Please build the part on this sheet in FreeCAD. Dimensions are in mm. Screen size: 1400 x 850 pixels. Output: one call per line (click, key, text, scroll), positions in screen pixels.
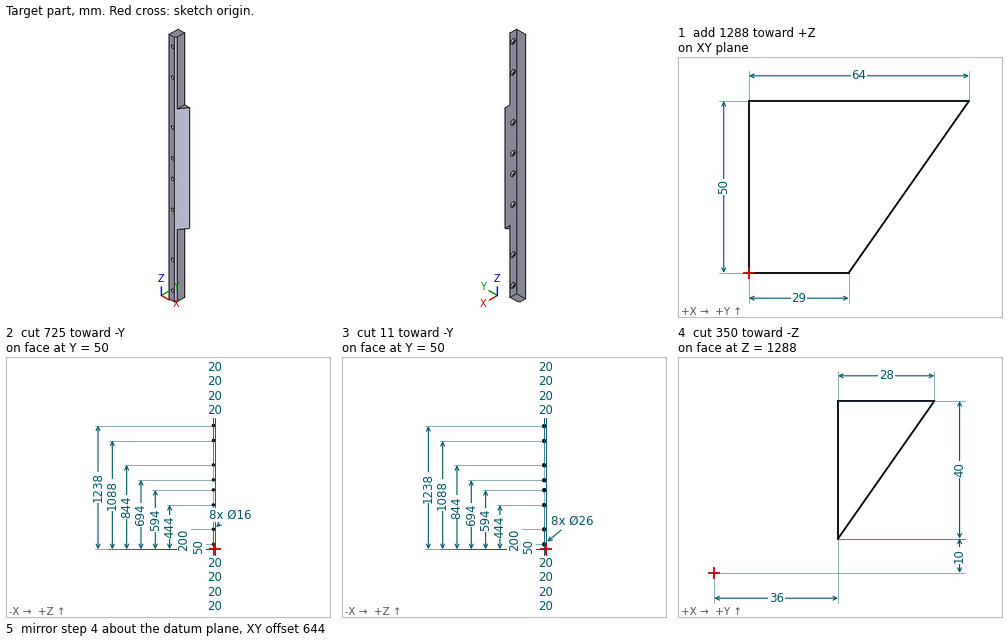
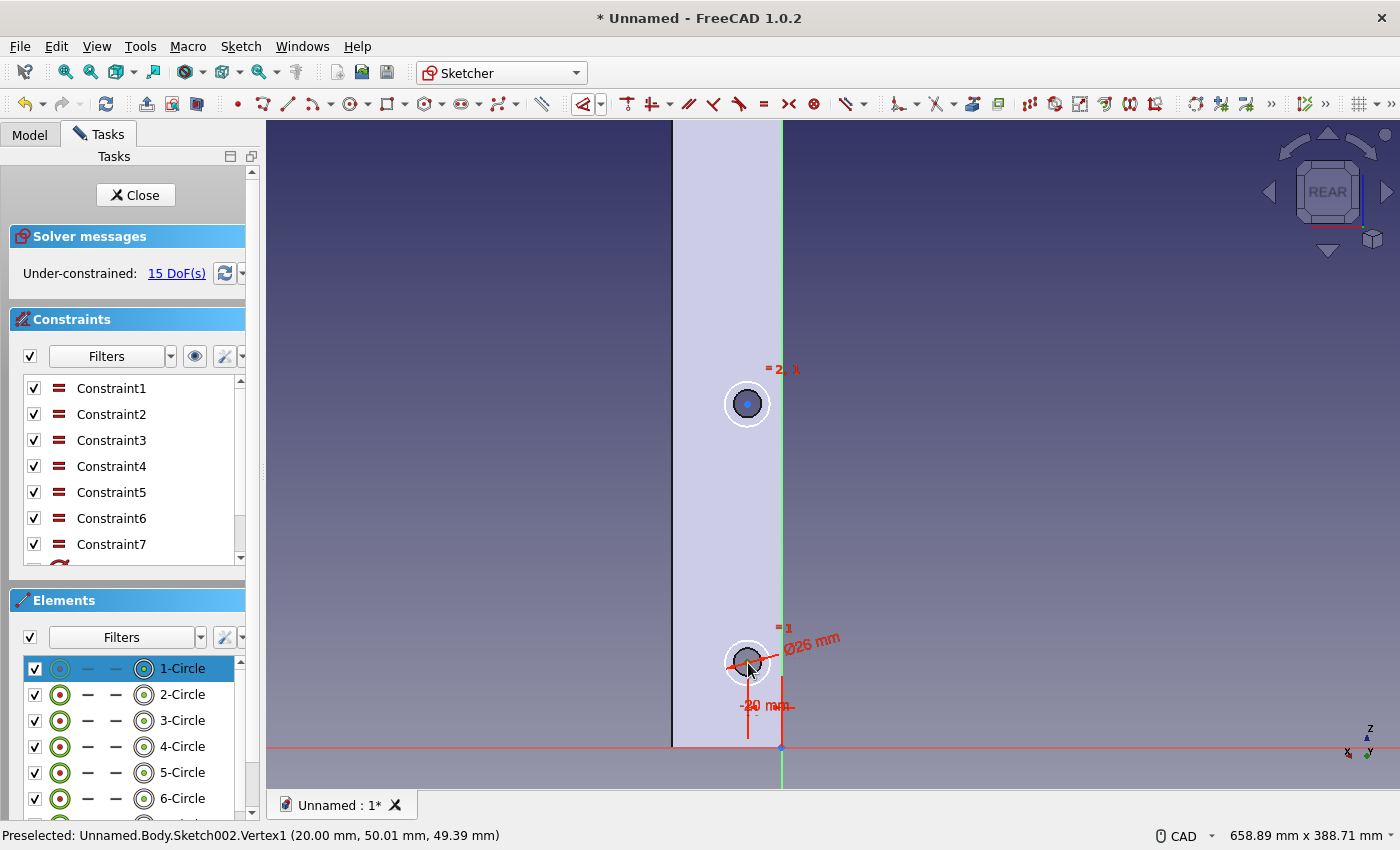
key(i)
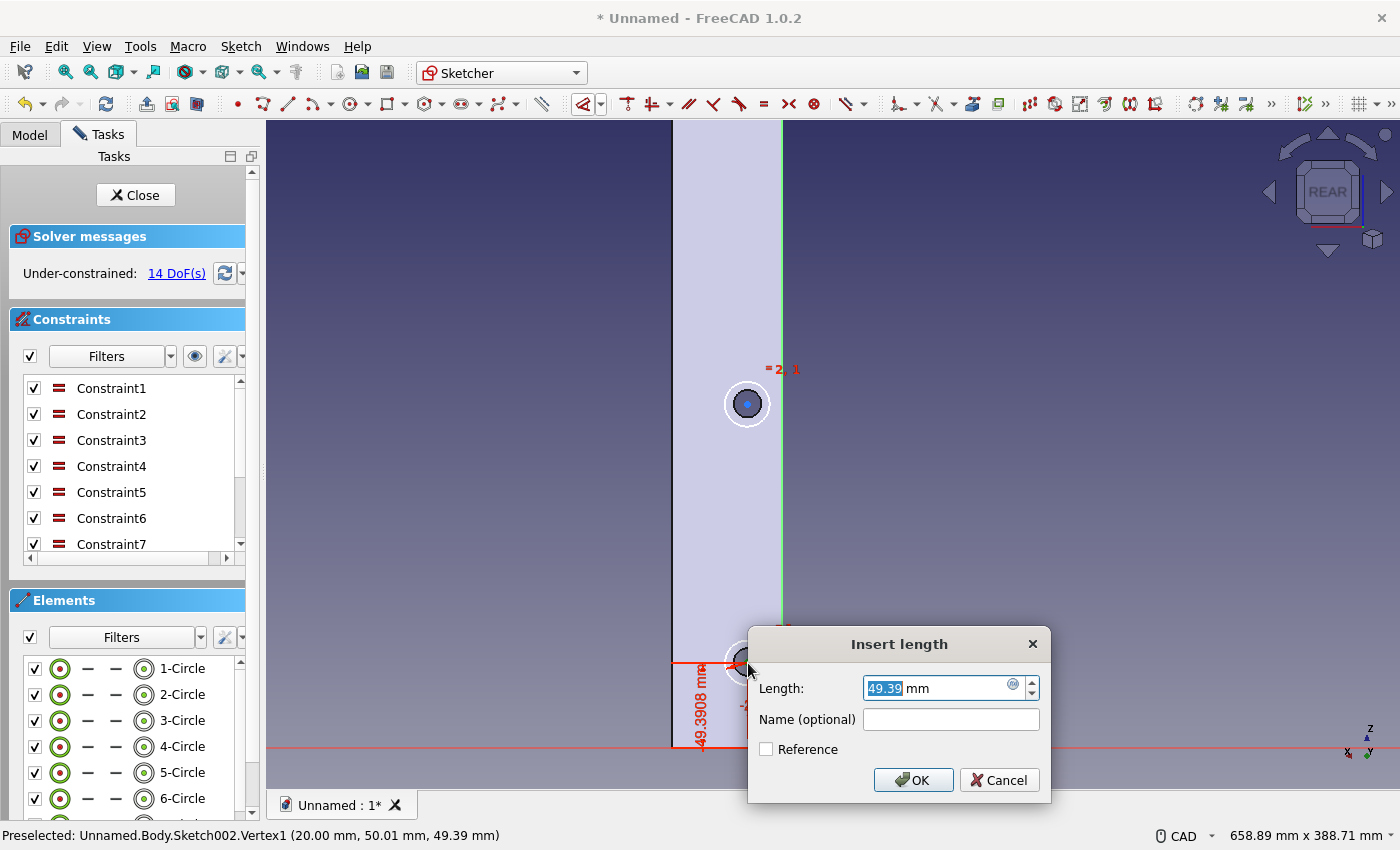
text(50)
key(Return)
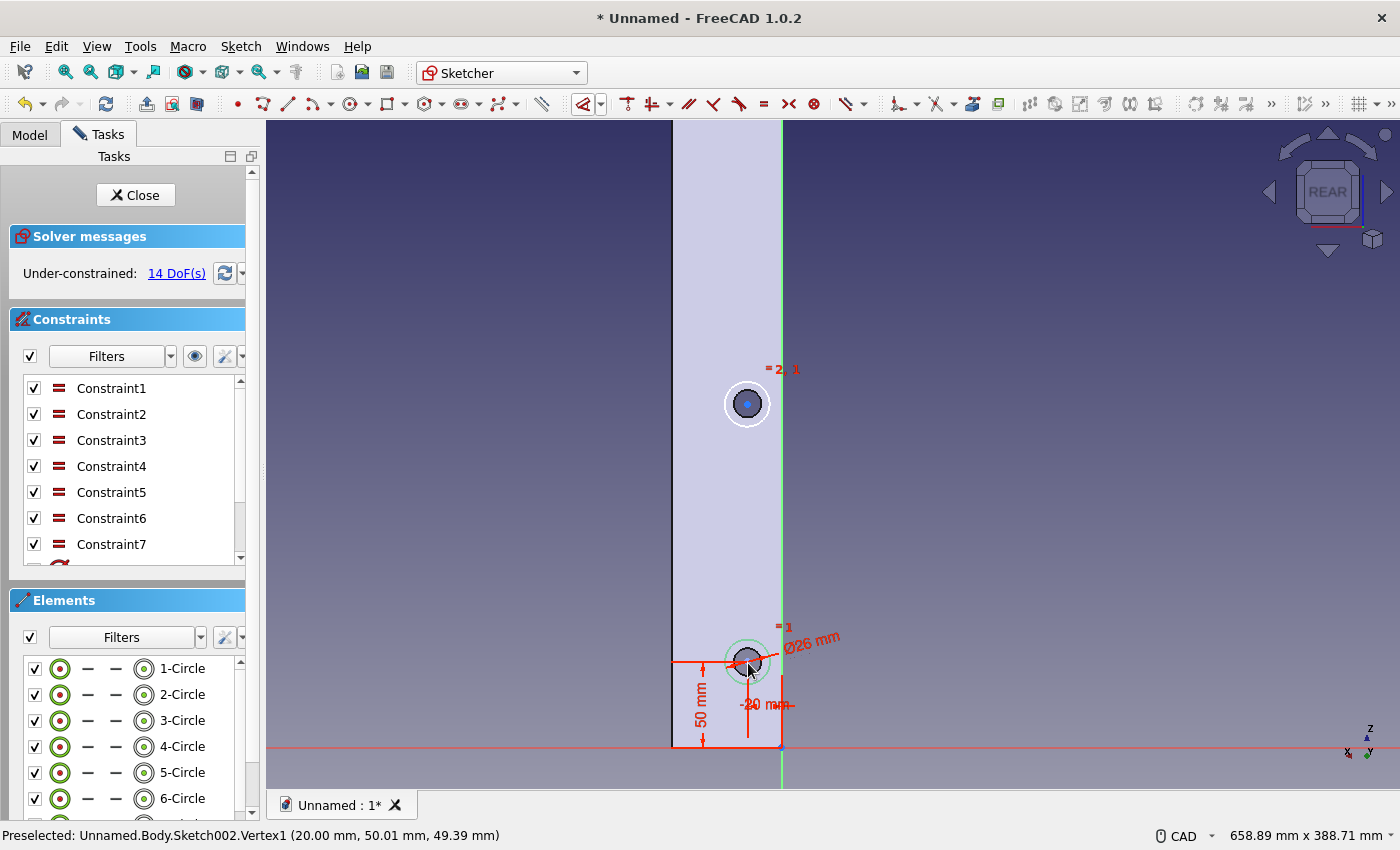
click(747, 404)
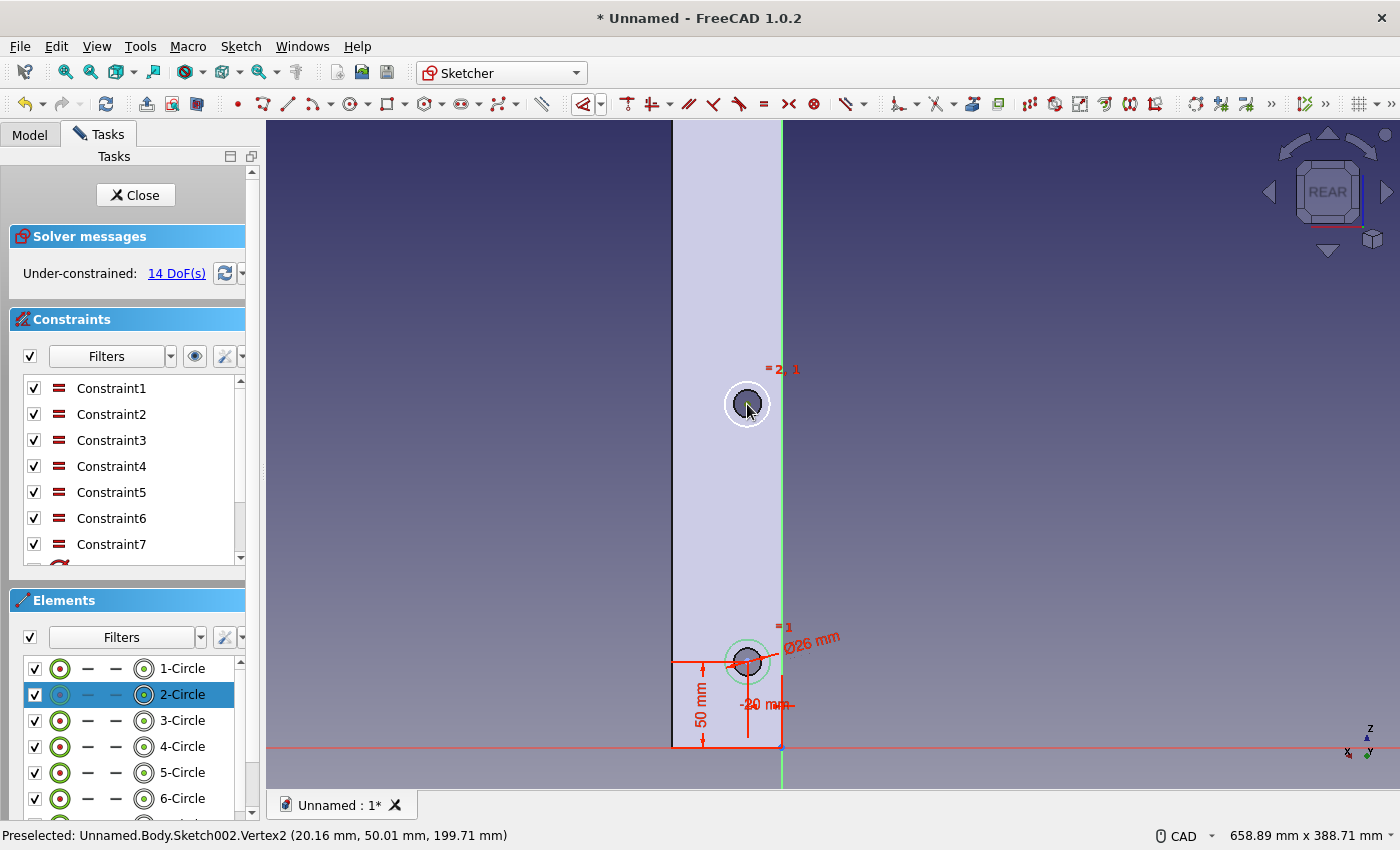
key(l)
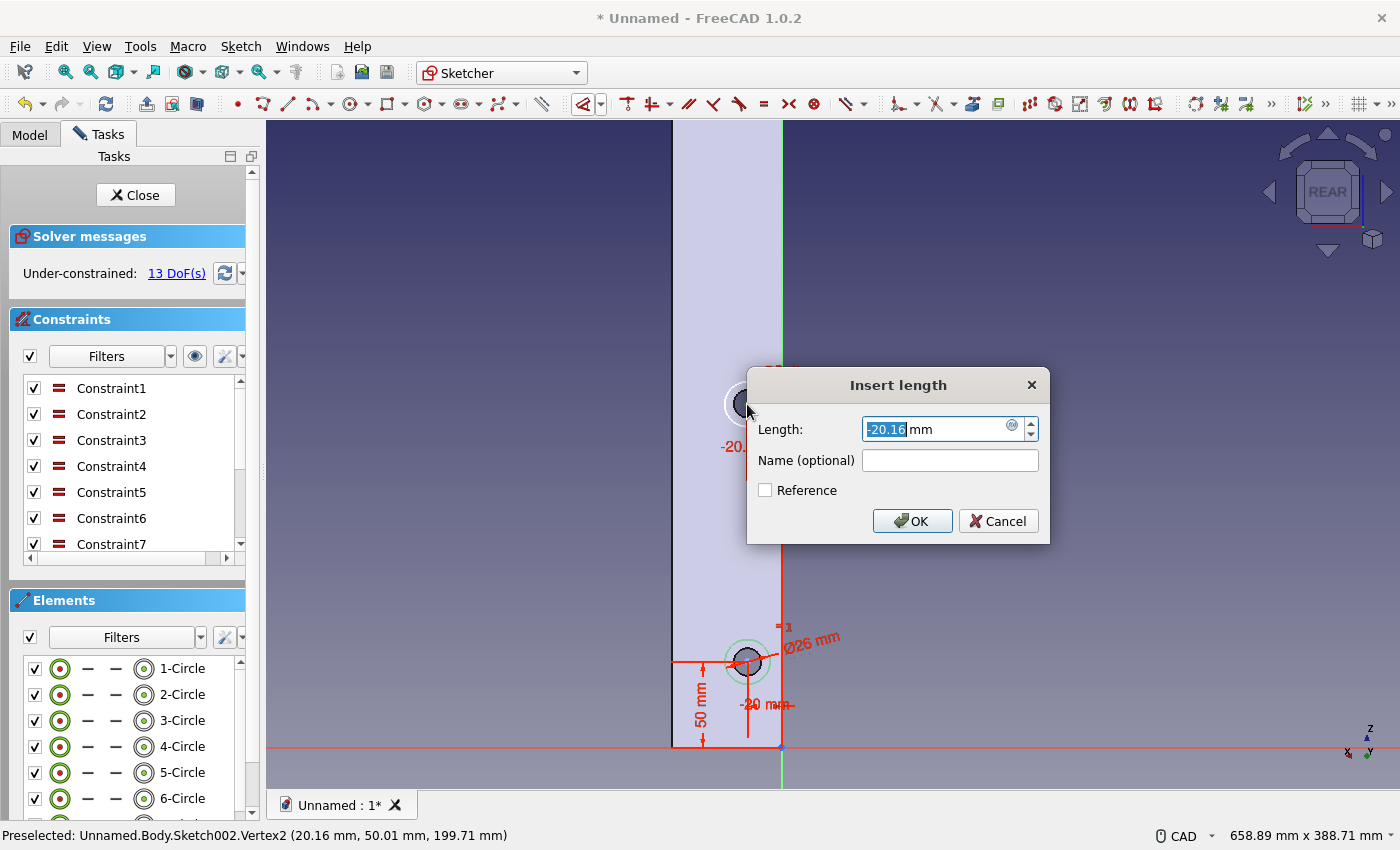
text(-20)
key(Return)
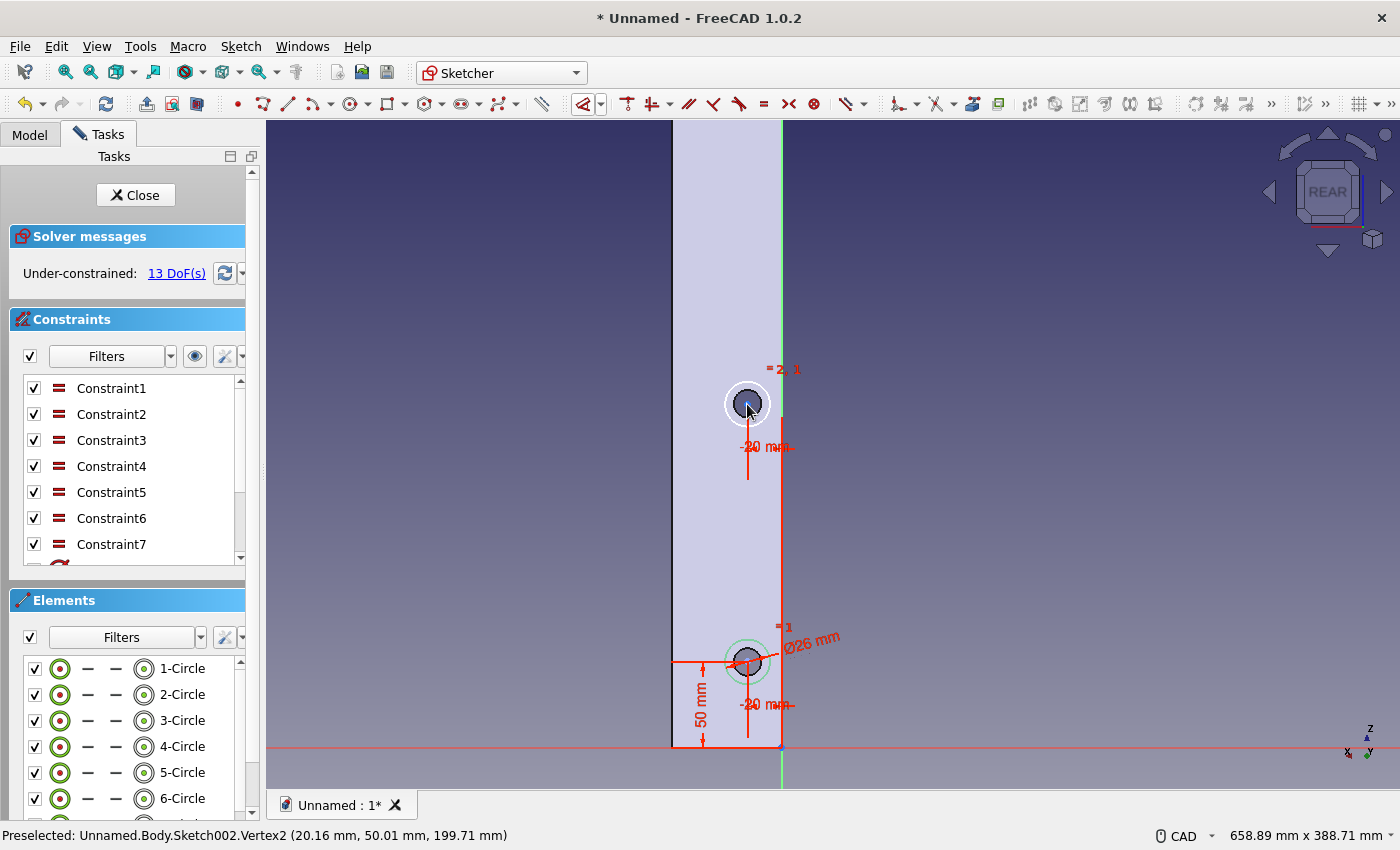
scroll(767, 653, down, 8)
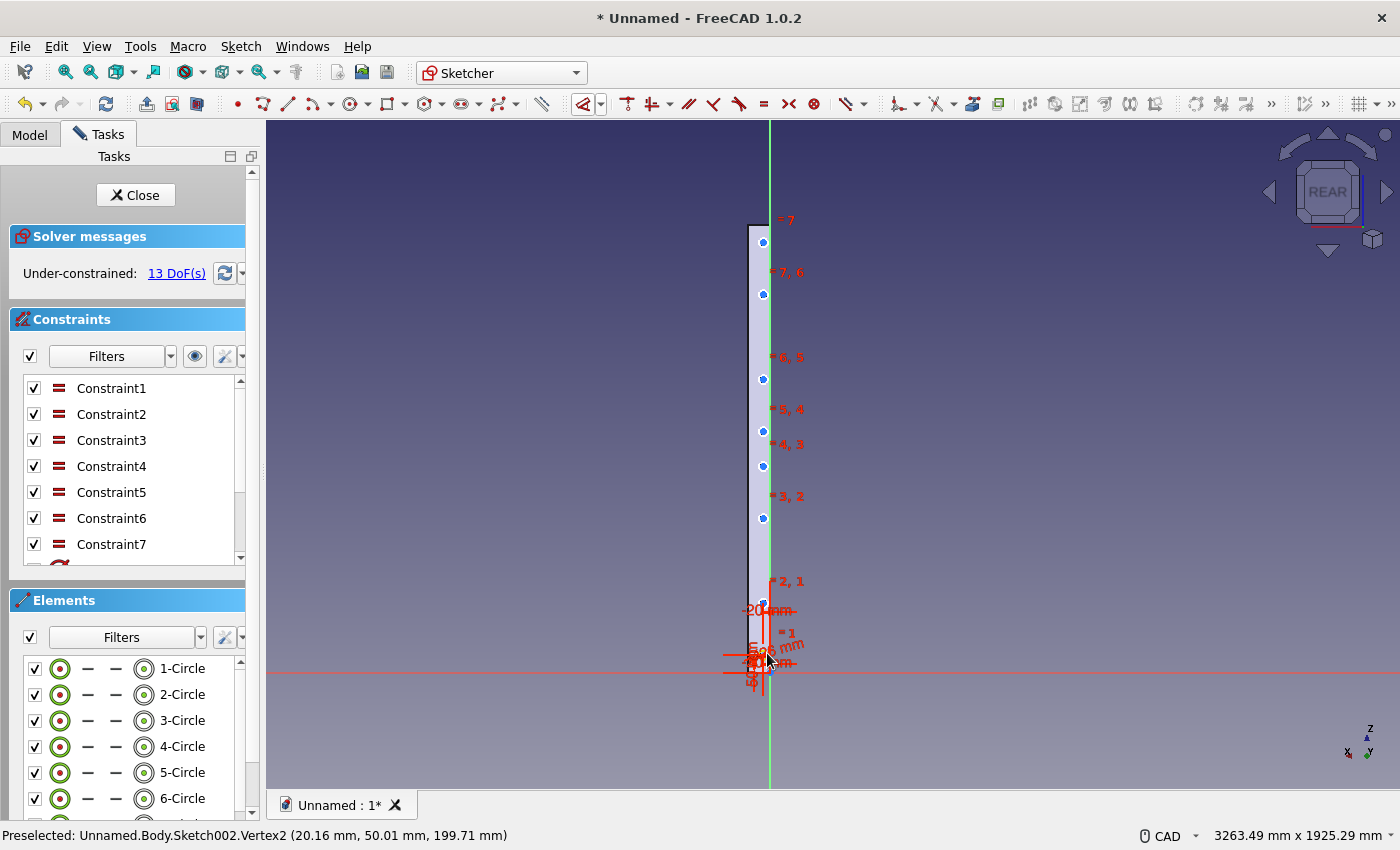
scroll(763, 519, up, 9)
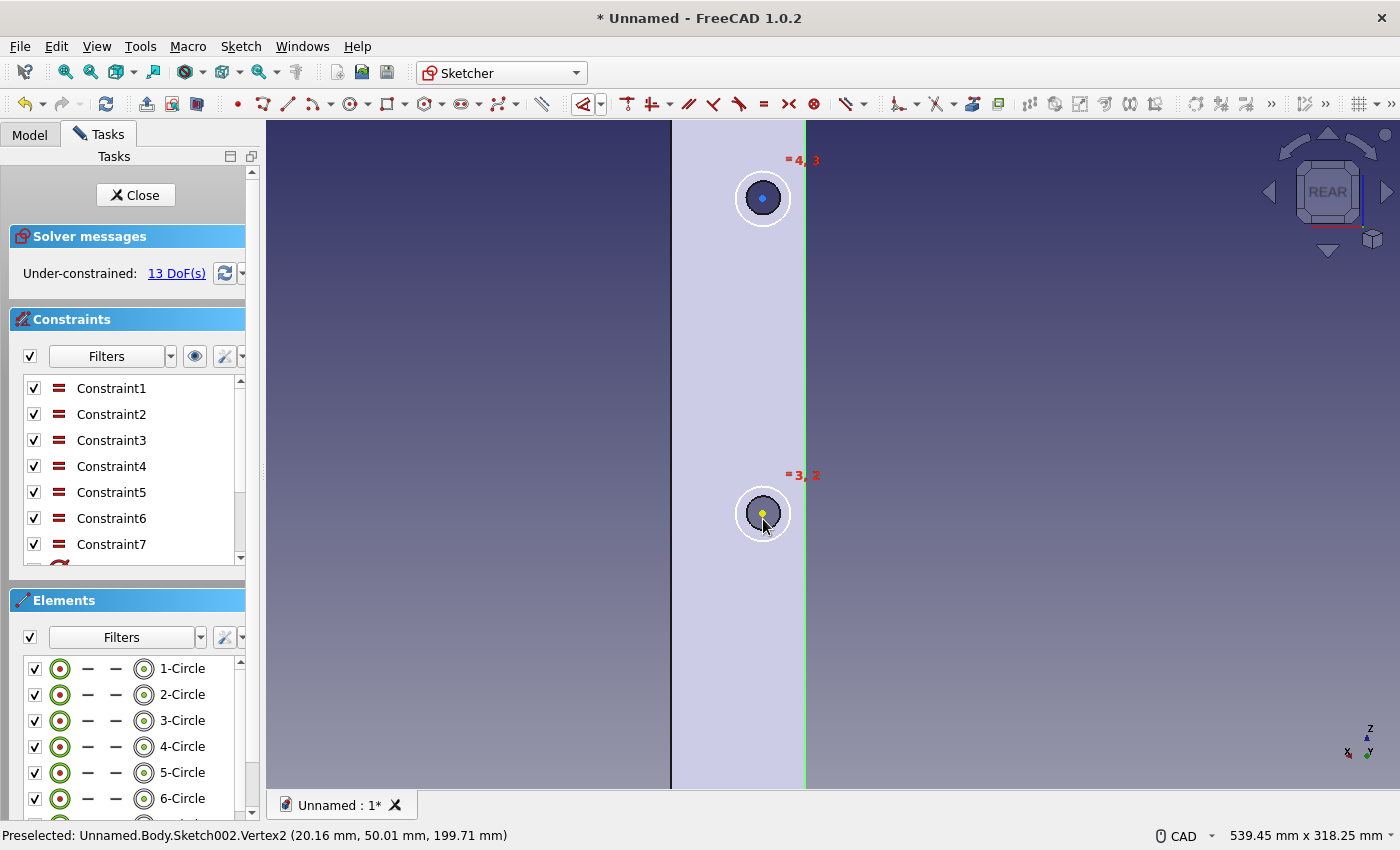
click(763, 514)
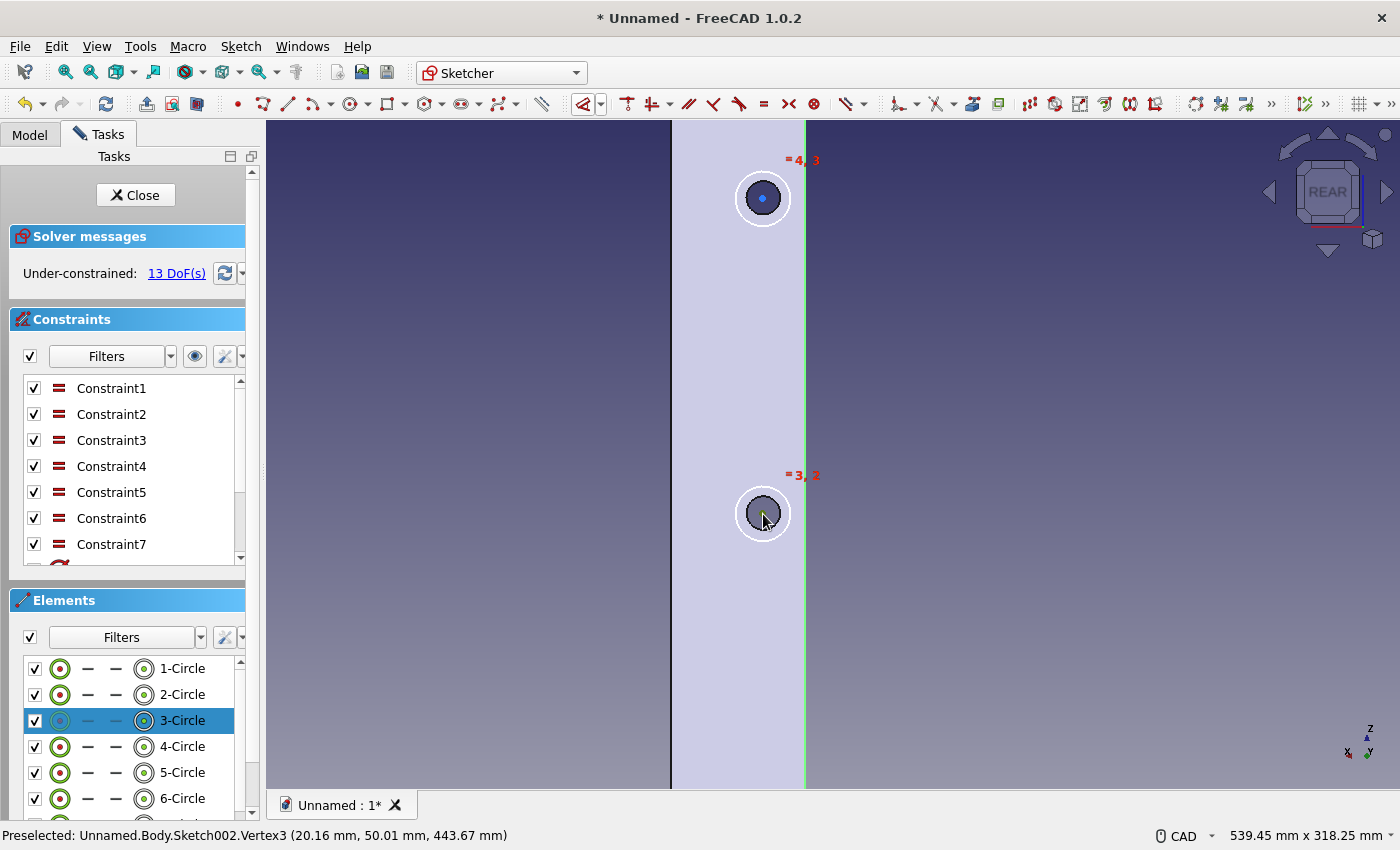
key(l)